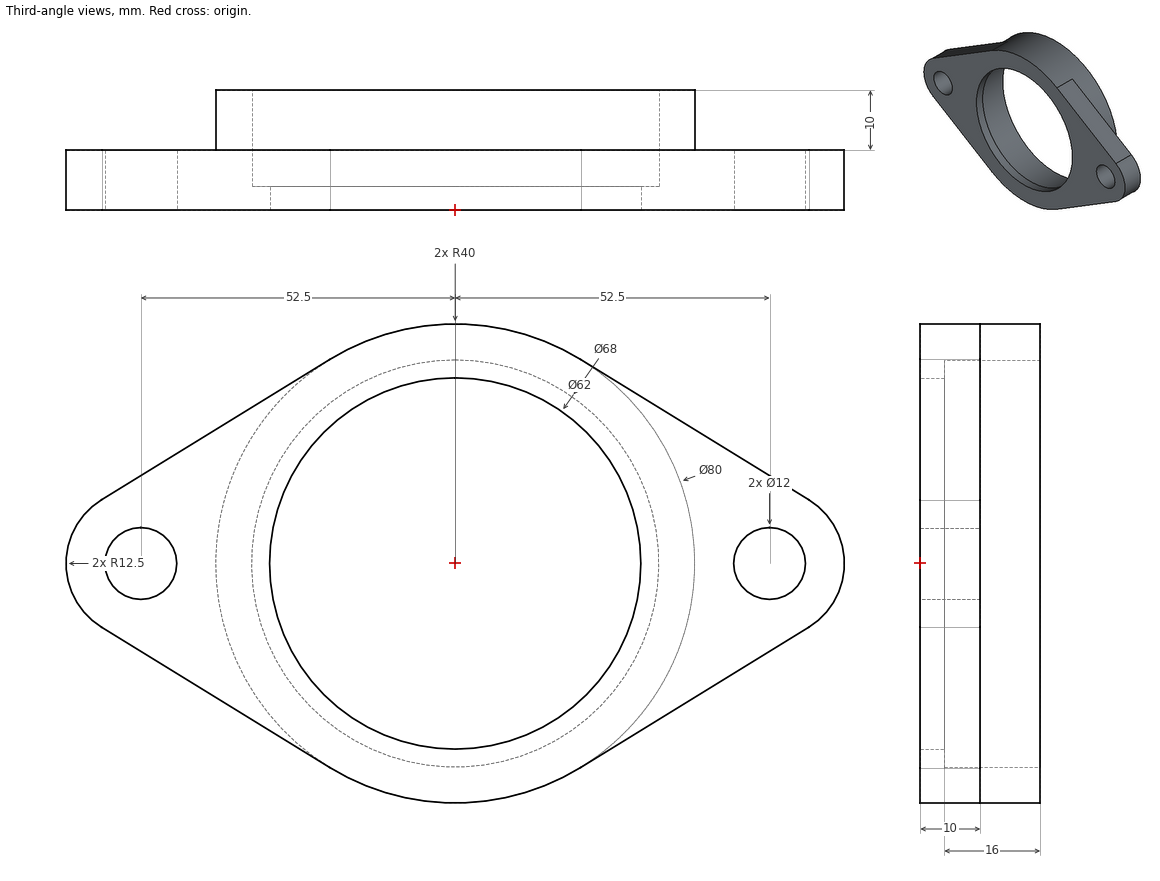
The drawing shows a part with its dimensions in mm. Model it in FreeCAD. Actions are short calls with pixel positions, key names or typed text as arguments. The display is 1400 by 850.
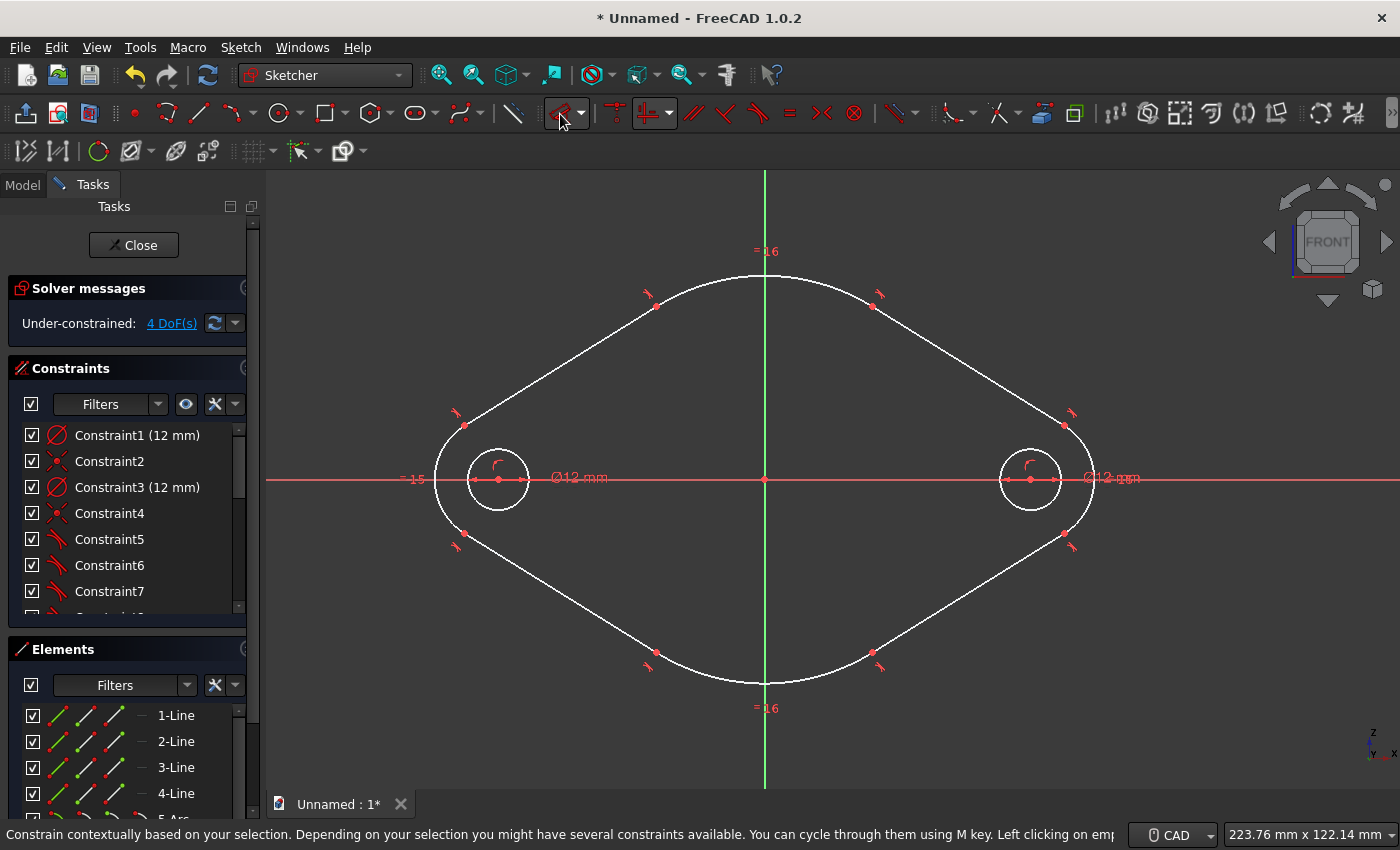
click(440, 455)
click(411, 443)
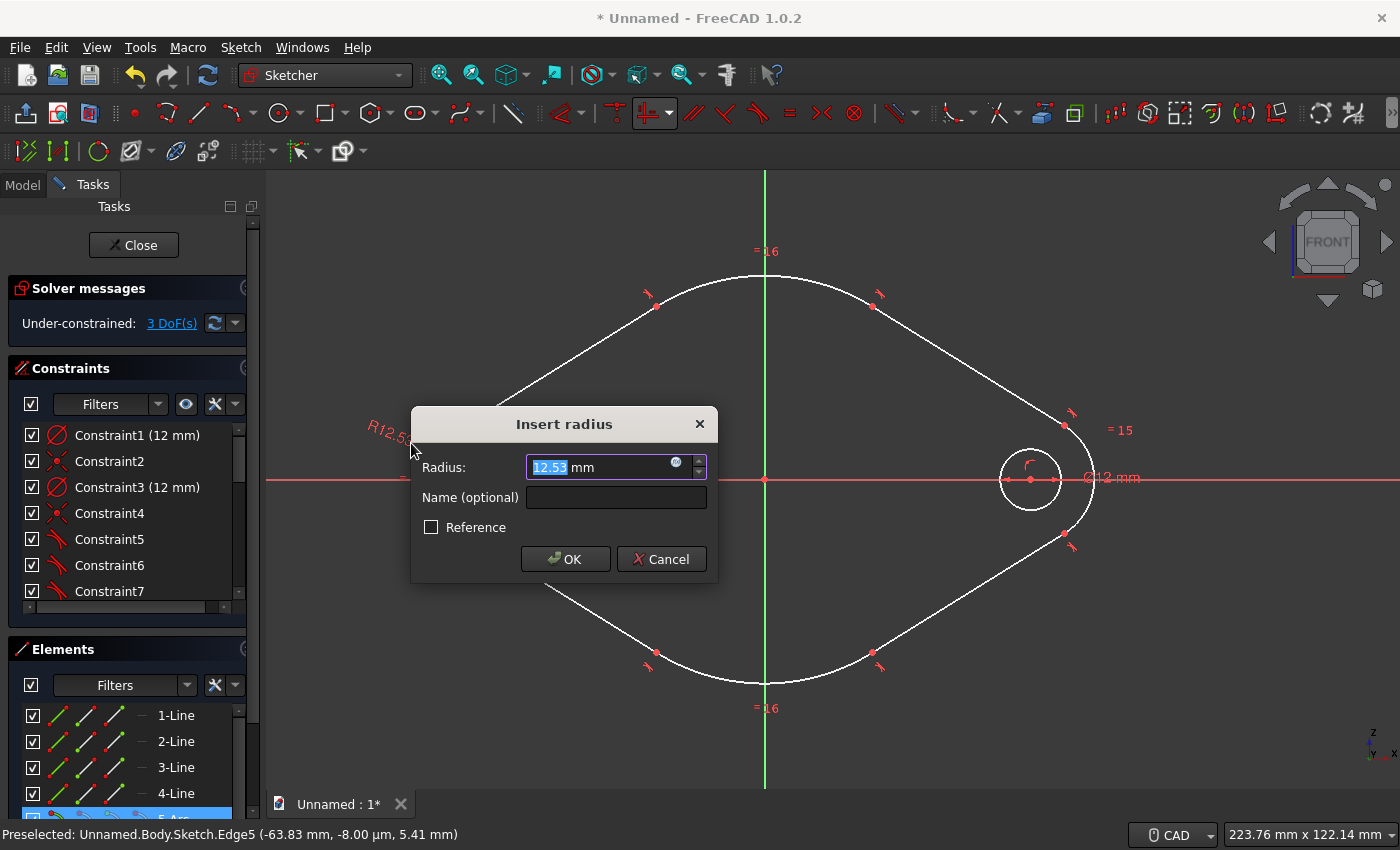
text(12.5)
key(Return)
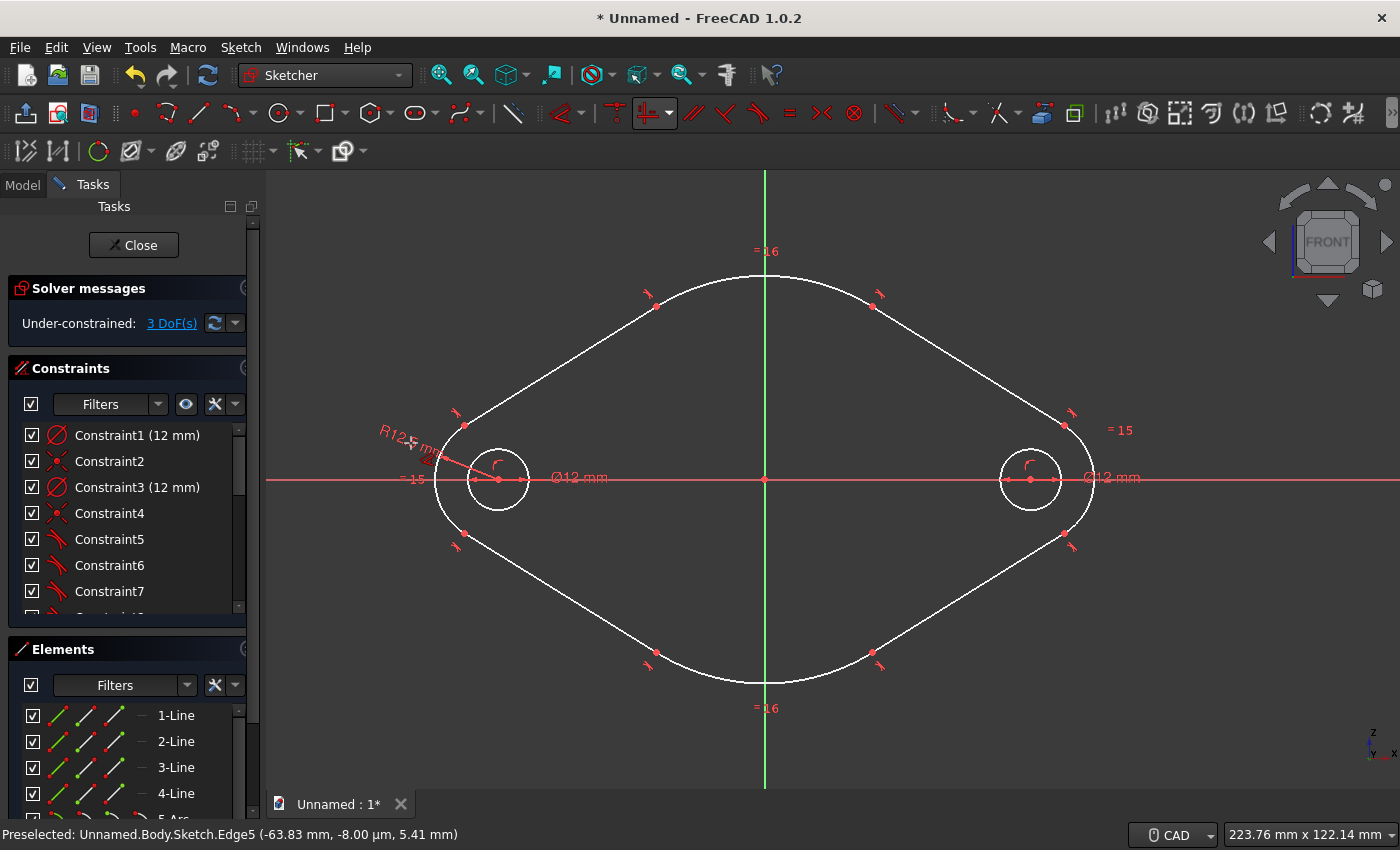
click(809, 281)
click(816, 250)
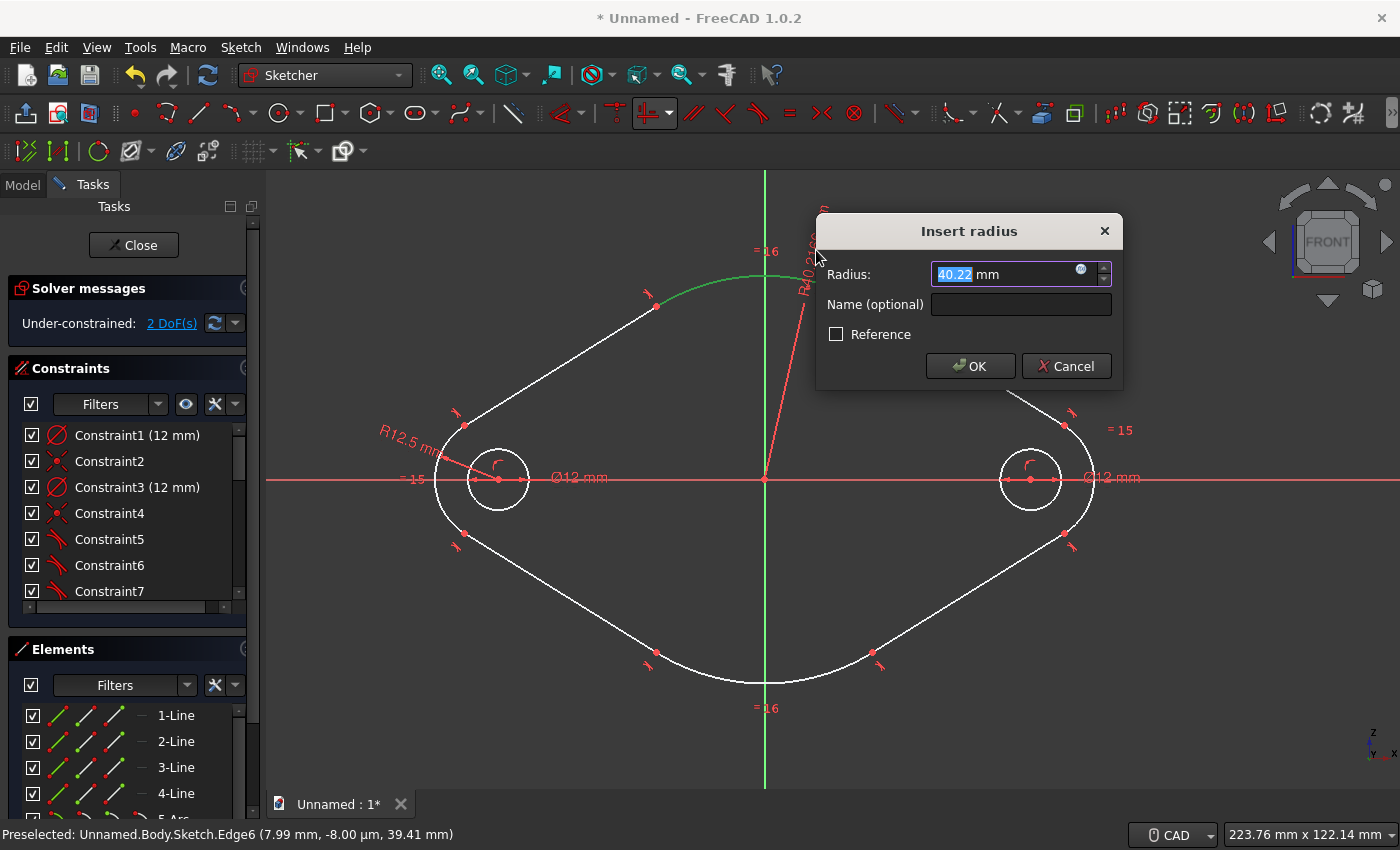
text(40)
key(Return)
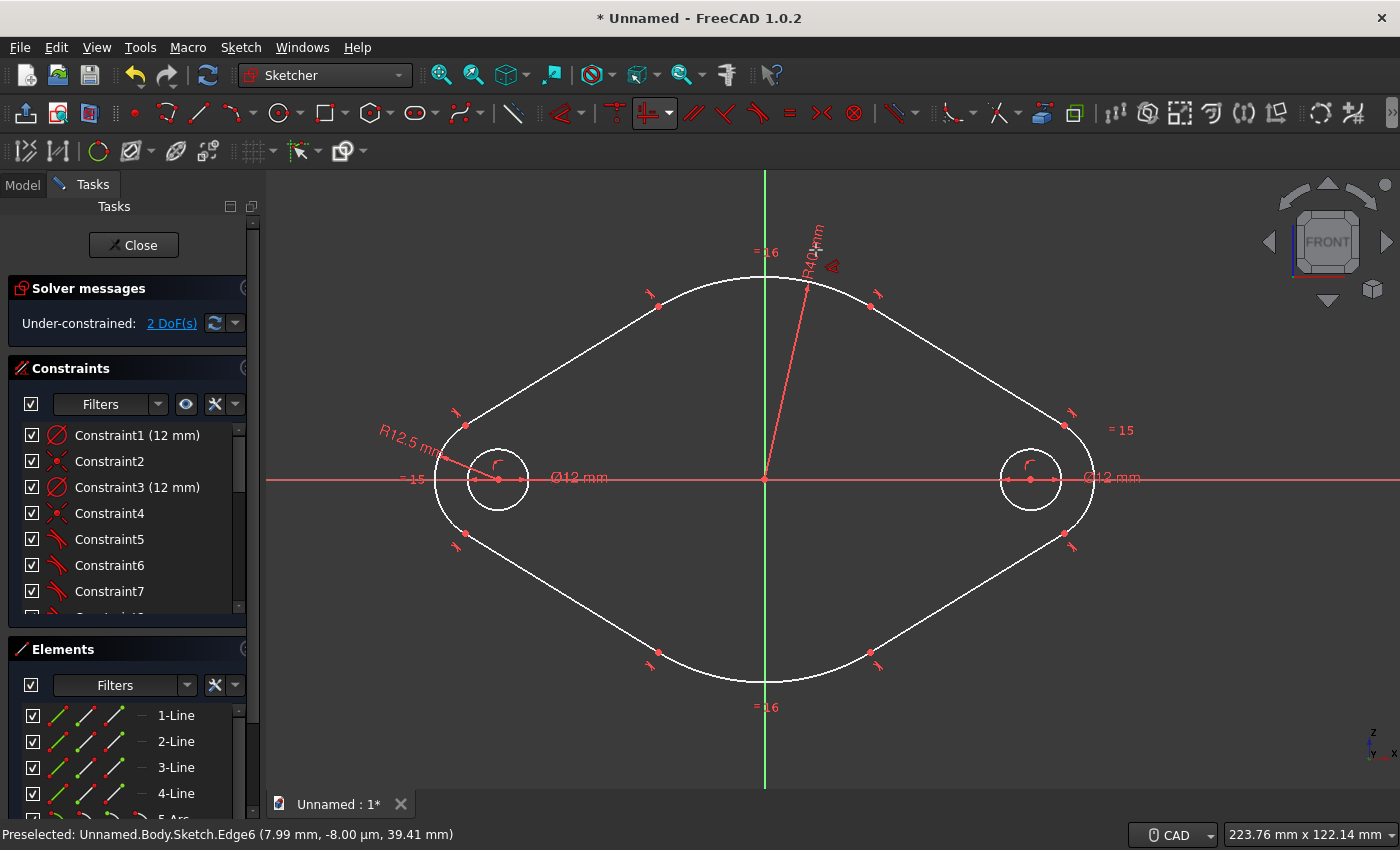
click(1031, 480)
click(898, 514)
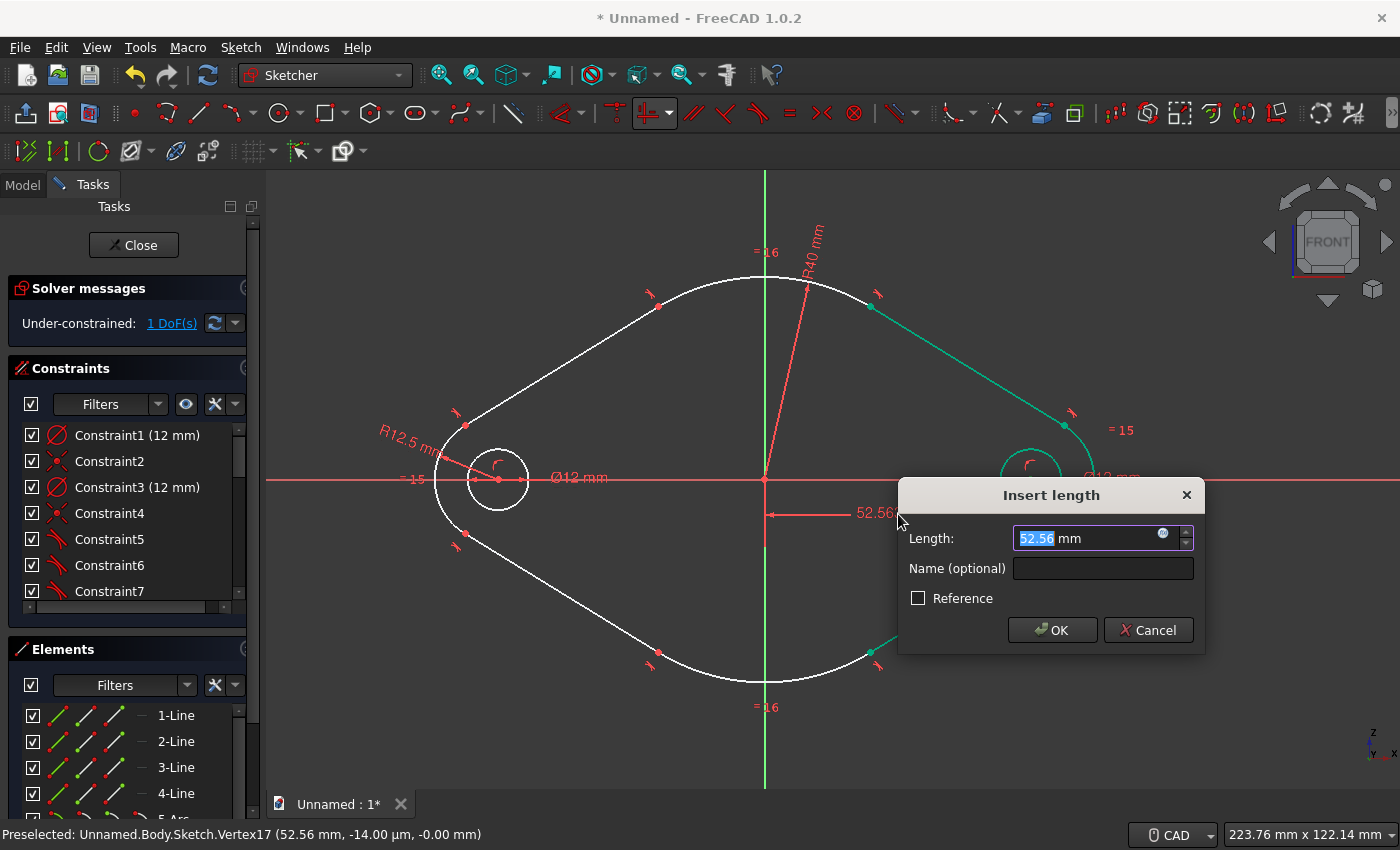
text(52.5)
key(Return)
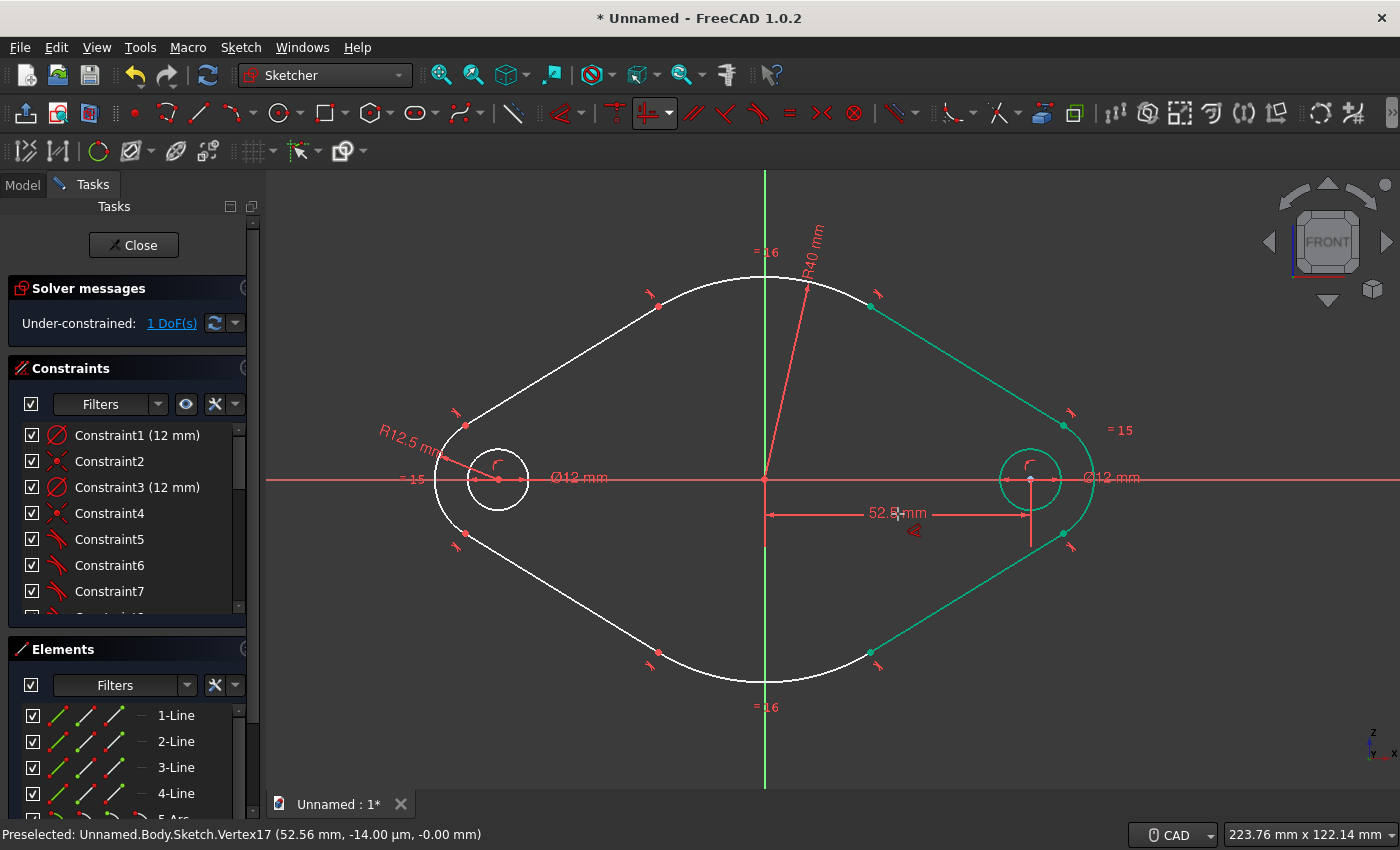
click(498, 480)
click(631, 514)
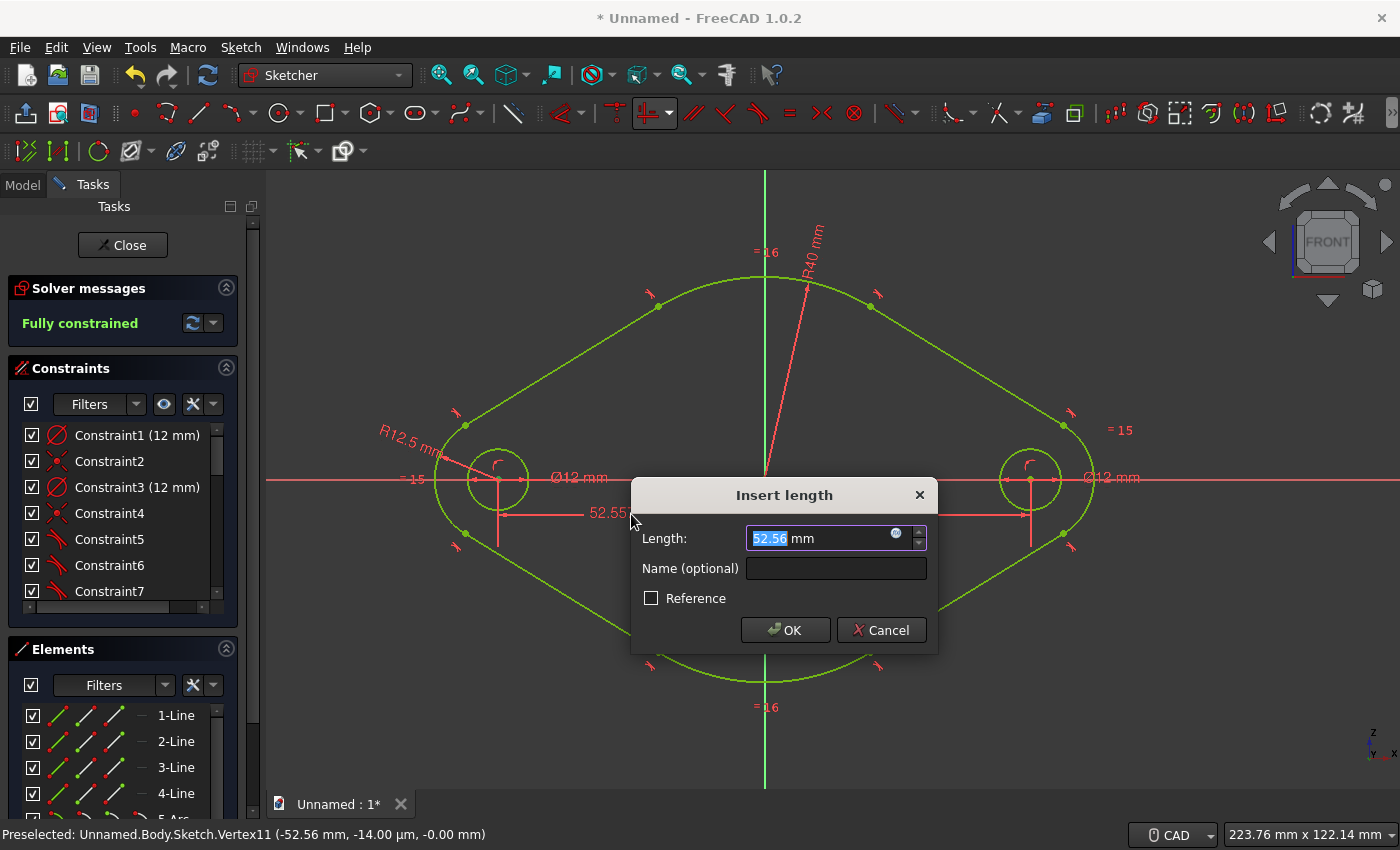
text(52.5)
key(Return)
key(Escape)